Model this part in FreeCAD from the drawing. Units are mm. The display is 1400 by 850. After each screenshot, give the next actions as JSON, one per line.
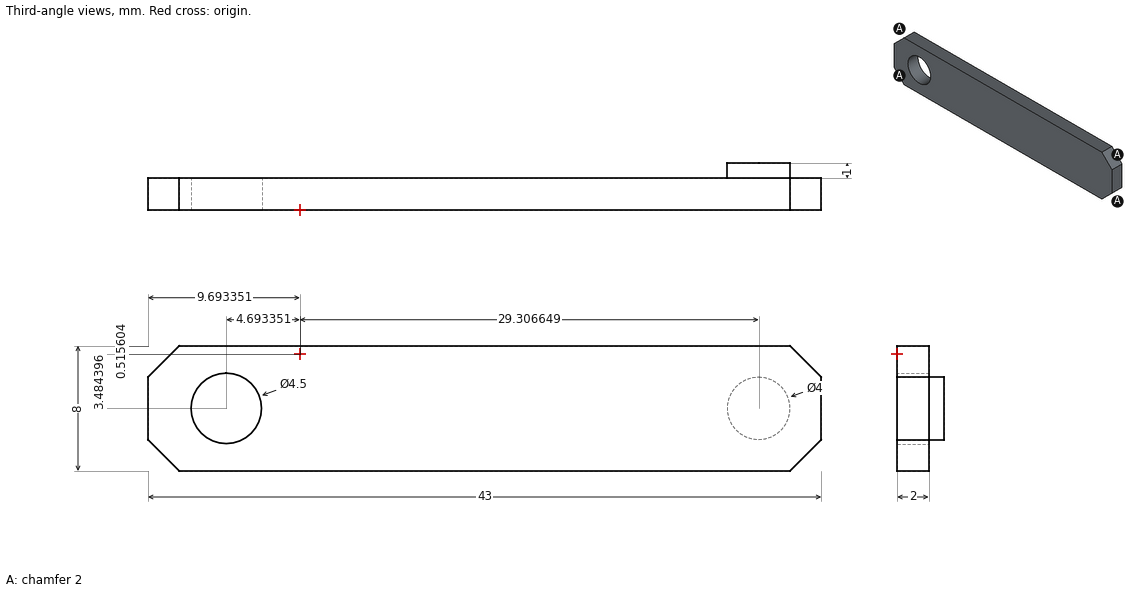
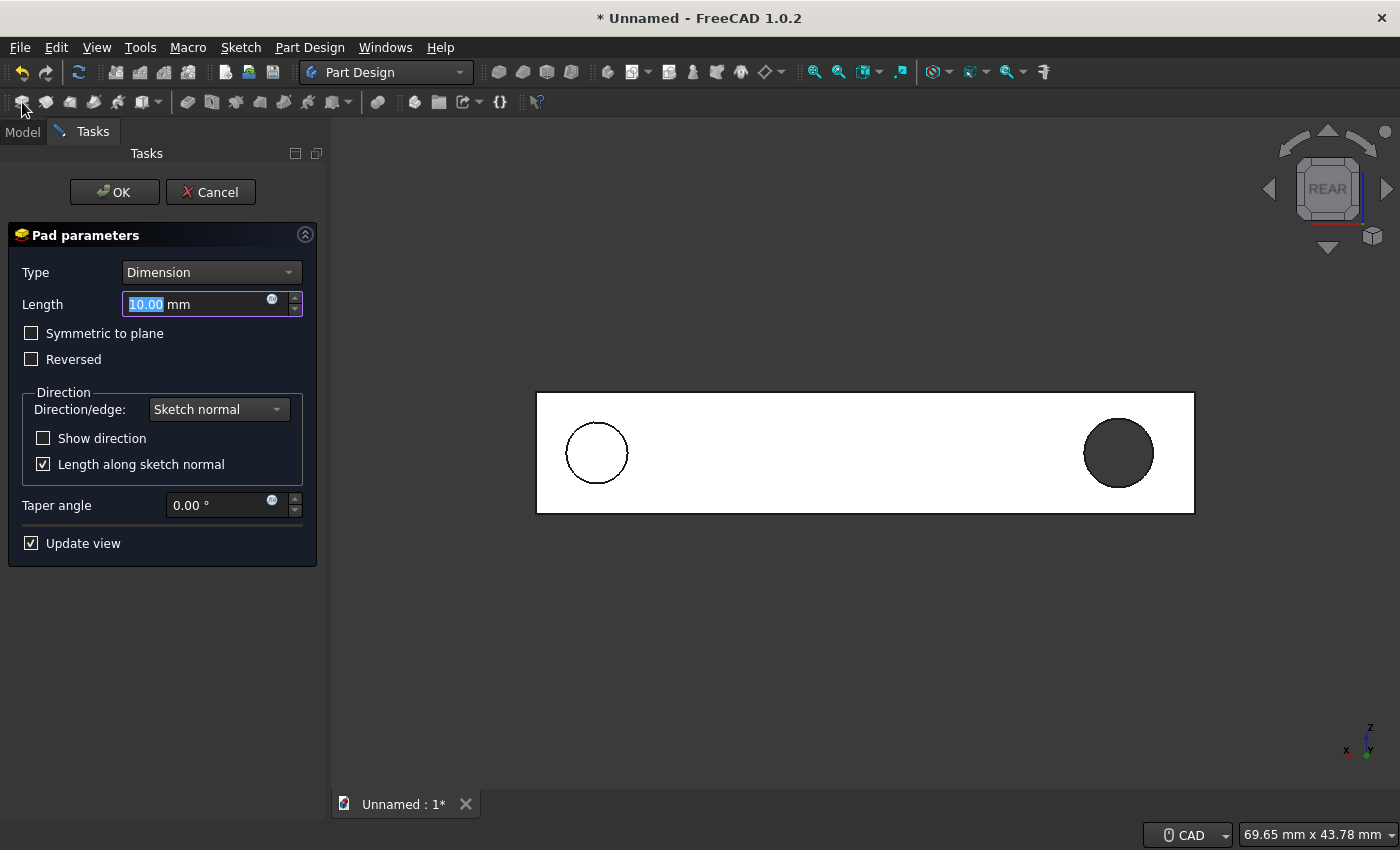
{"action": "type", "text": "1"}
{"action": "key", "text": "Tab"}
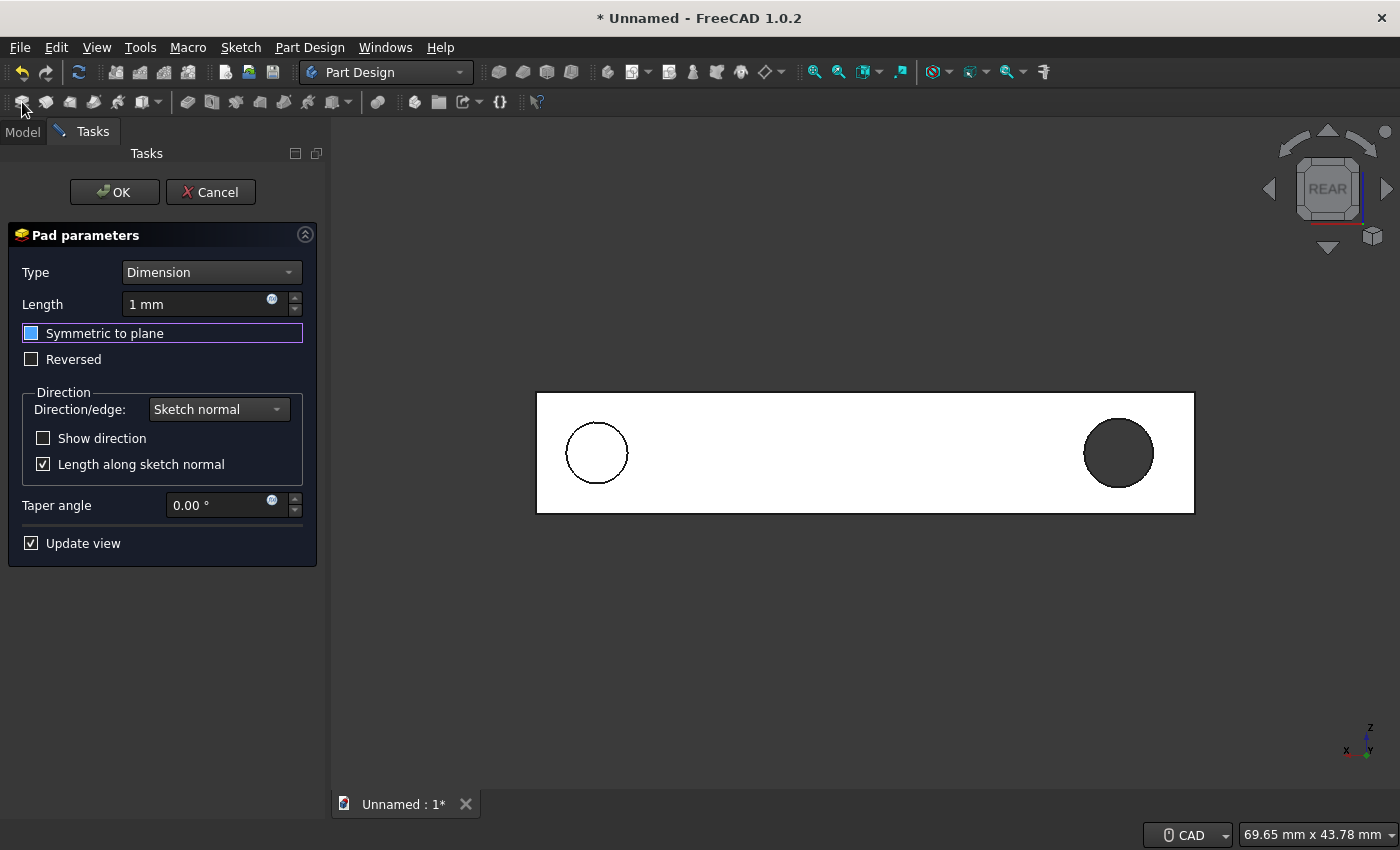
{"action": "left_click", "coordinate": [115, 192]}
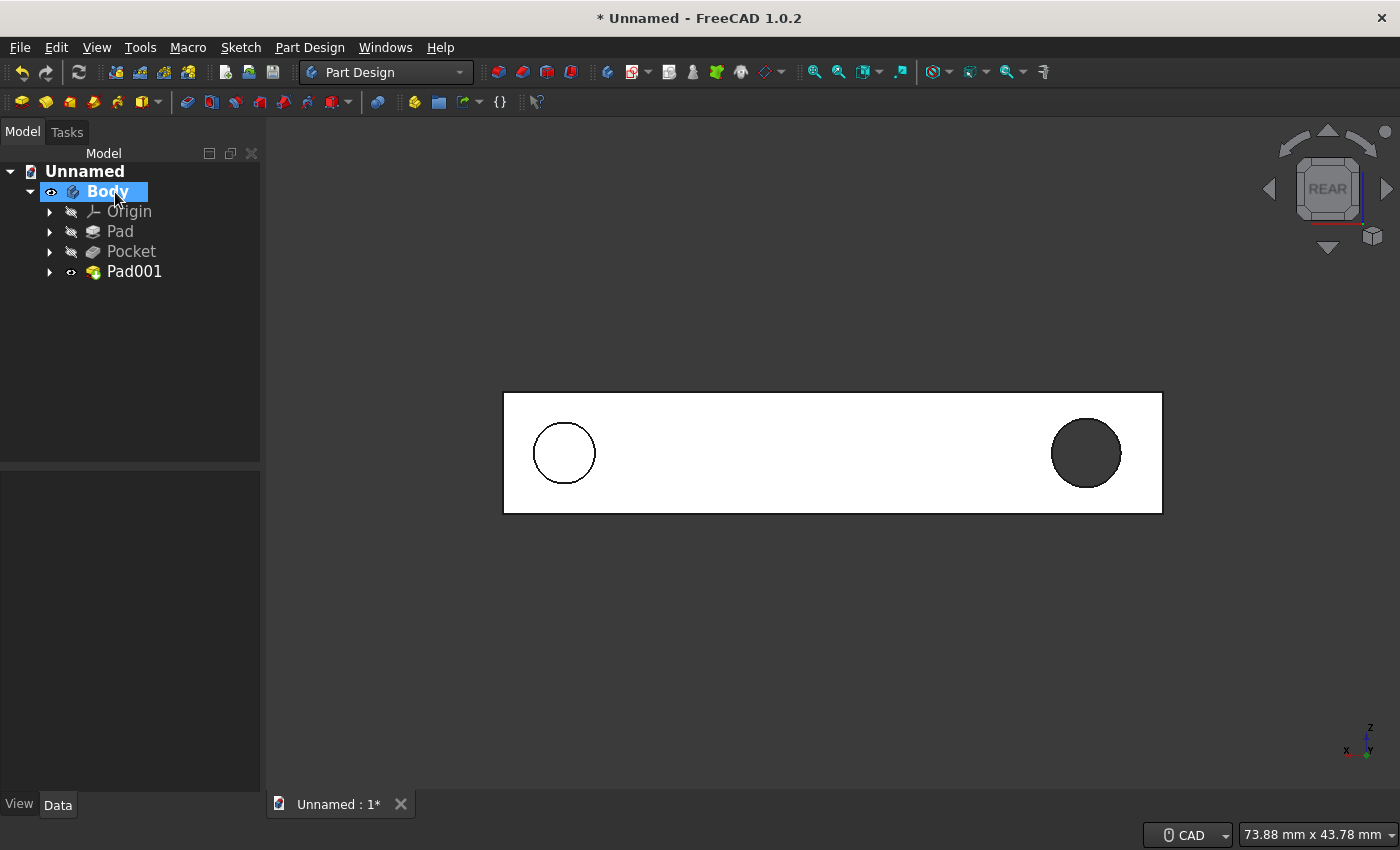
{"action": "key", "text": "0"}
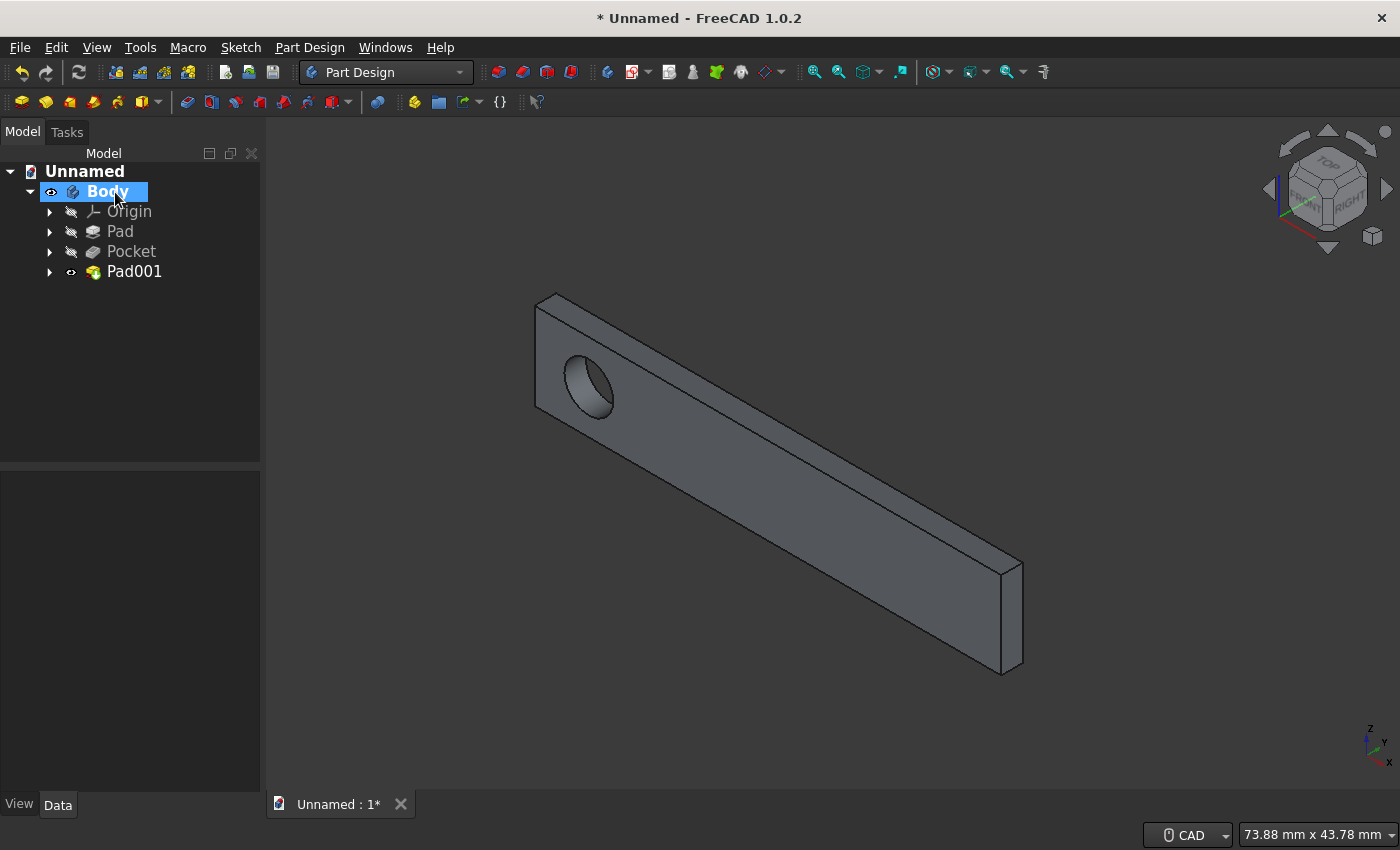
{"action": "left_click", "coordinate": [1012, 568]}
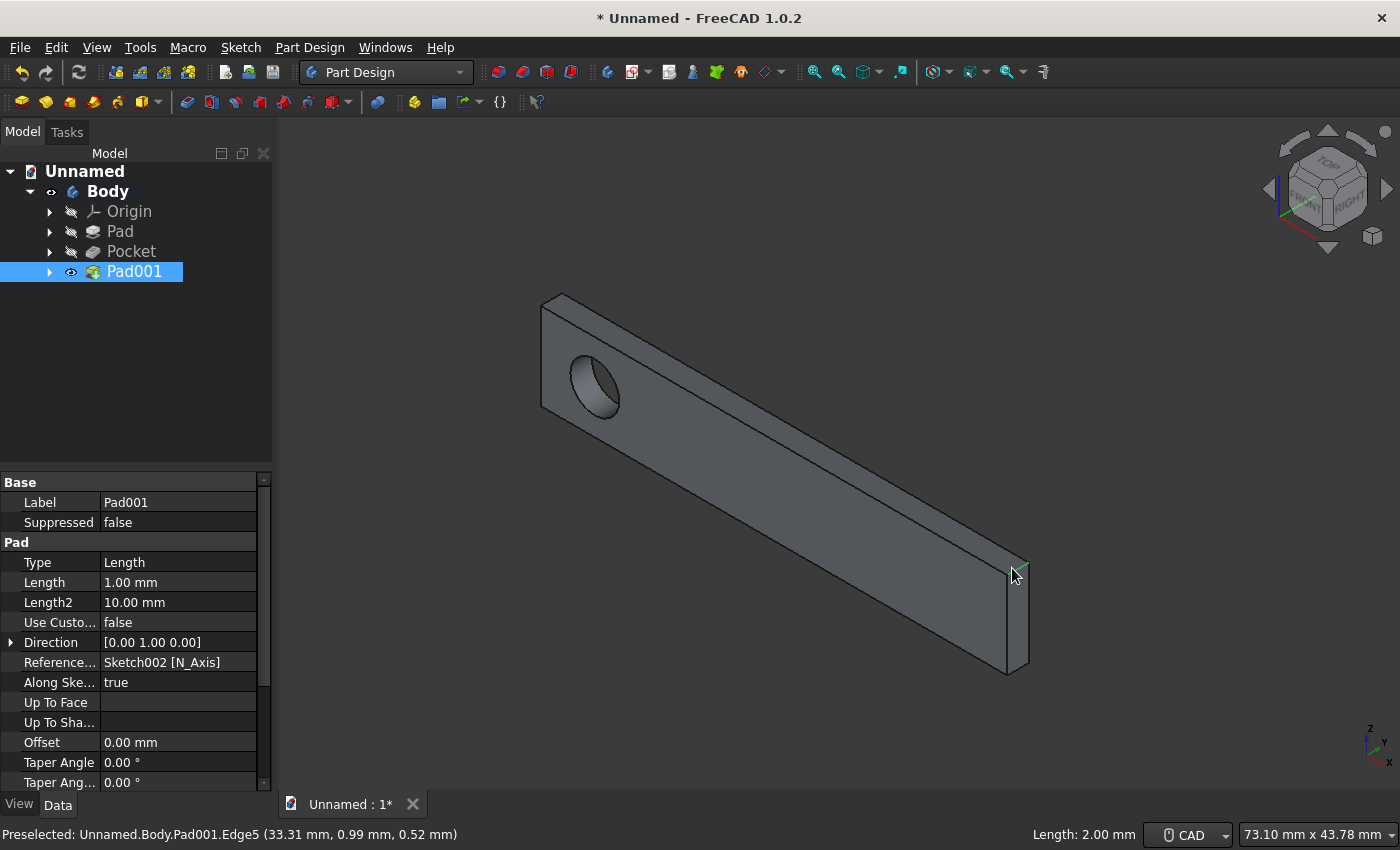
{"action": "key", "text": "2"}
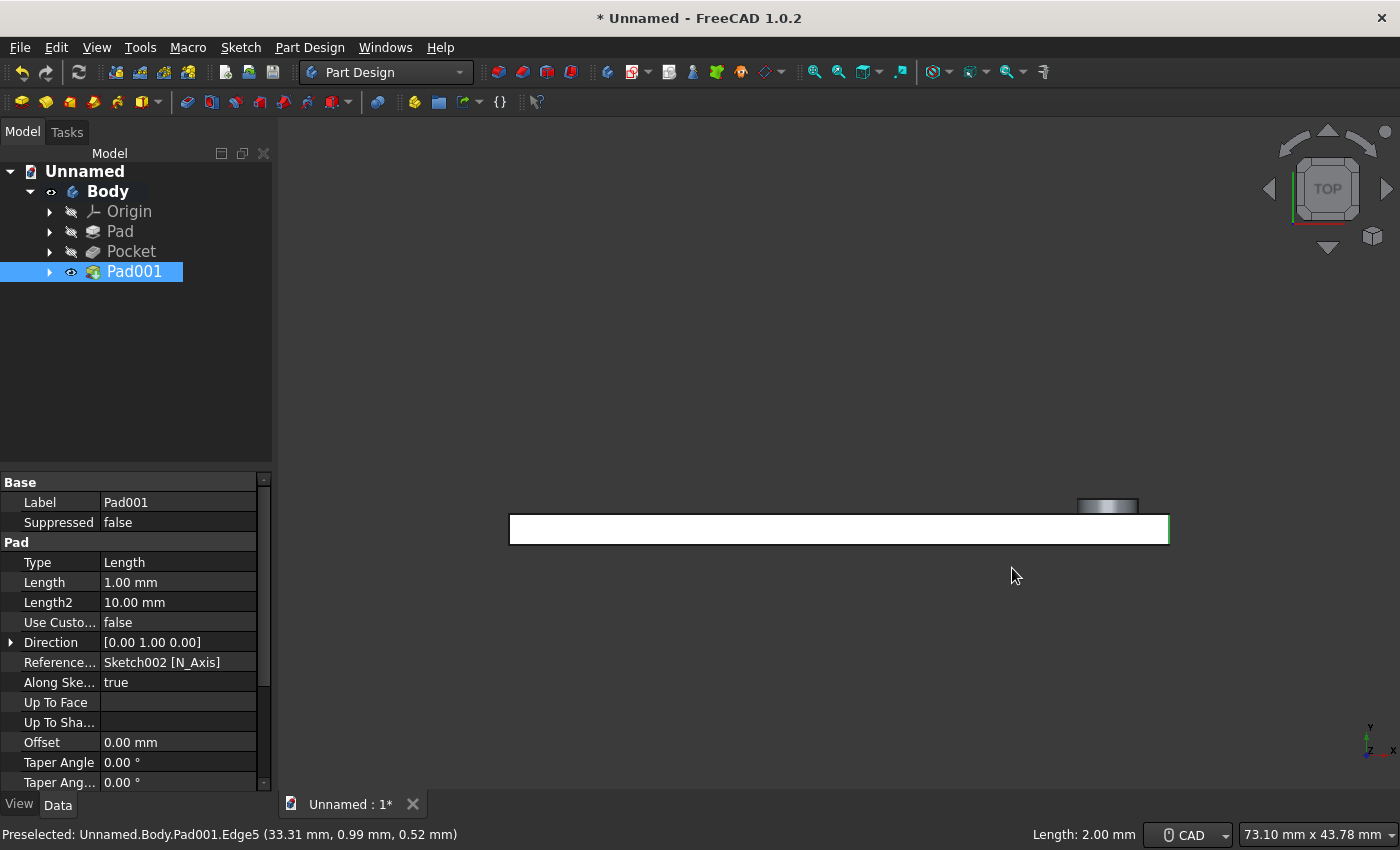
{"action": "left_click", "coordinate": [509, 529], "text": "ctrl"}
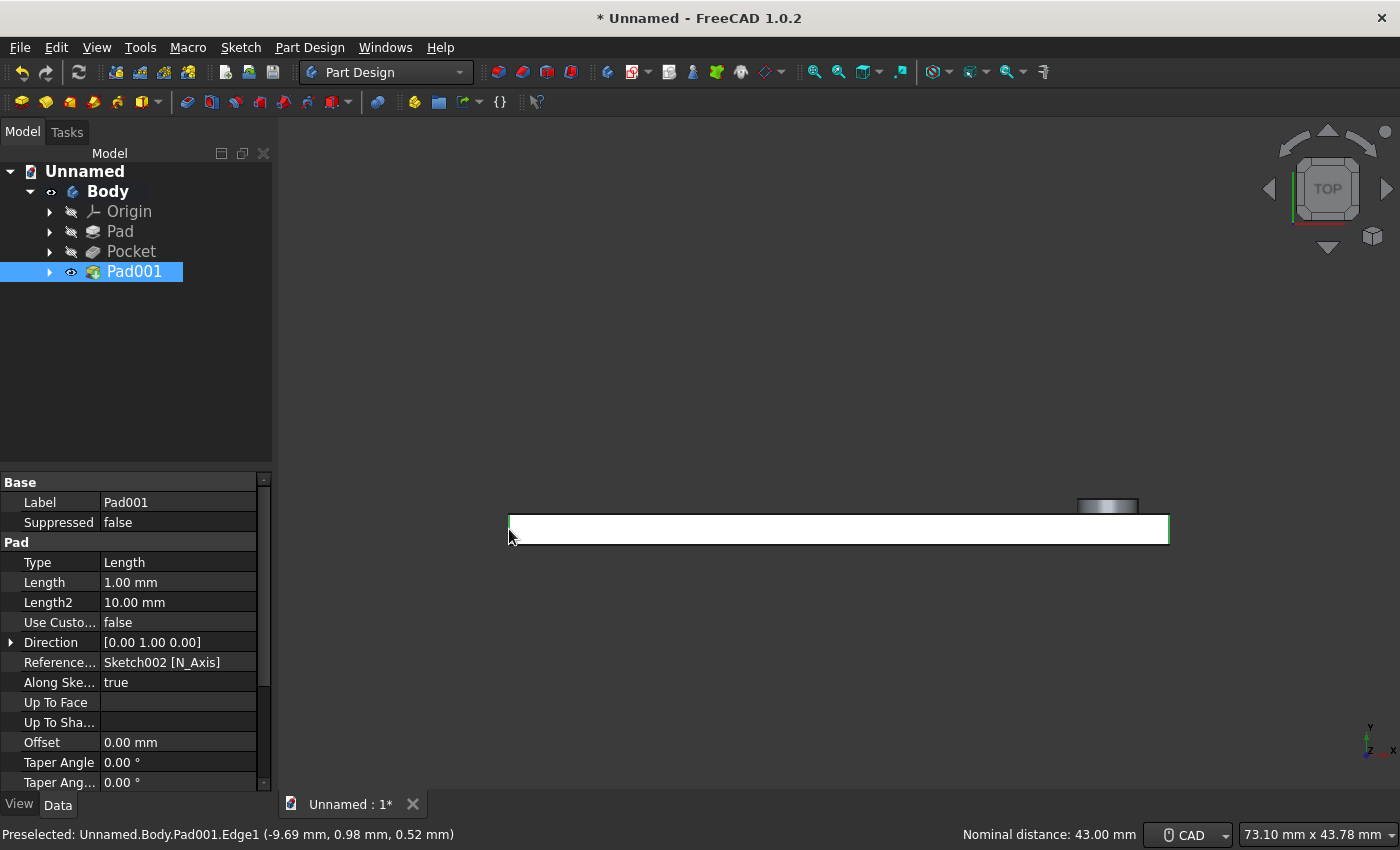
{"action": "key", "text": "1"}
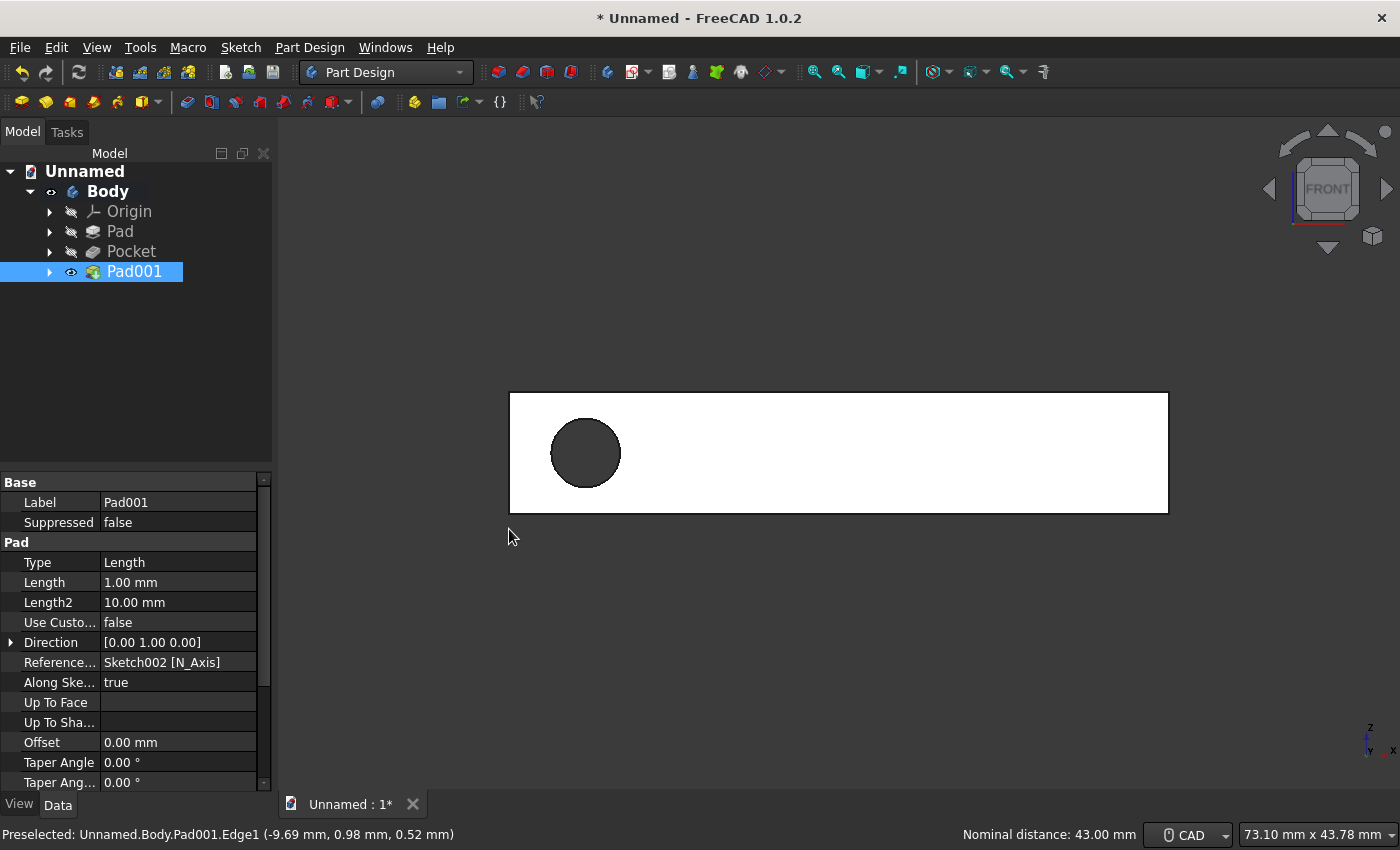
{"action": "key", "text": "3"}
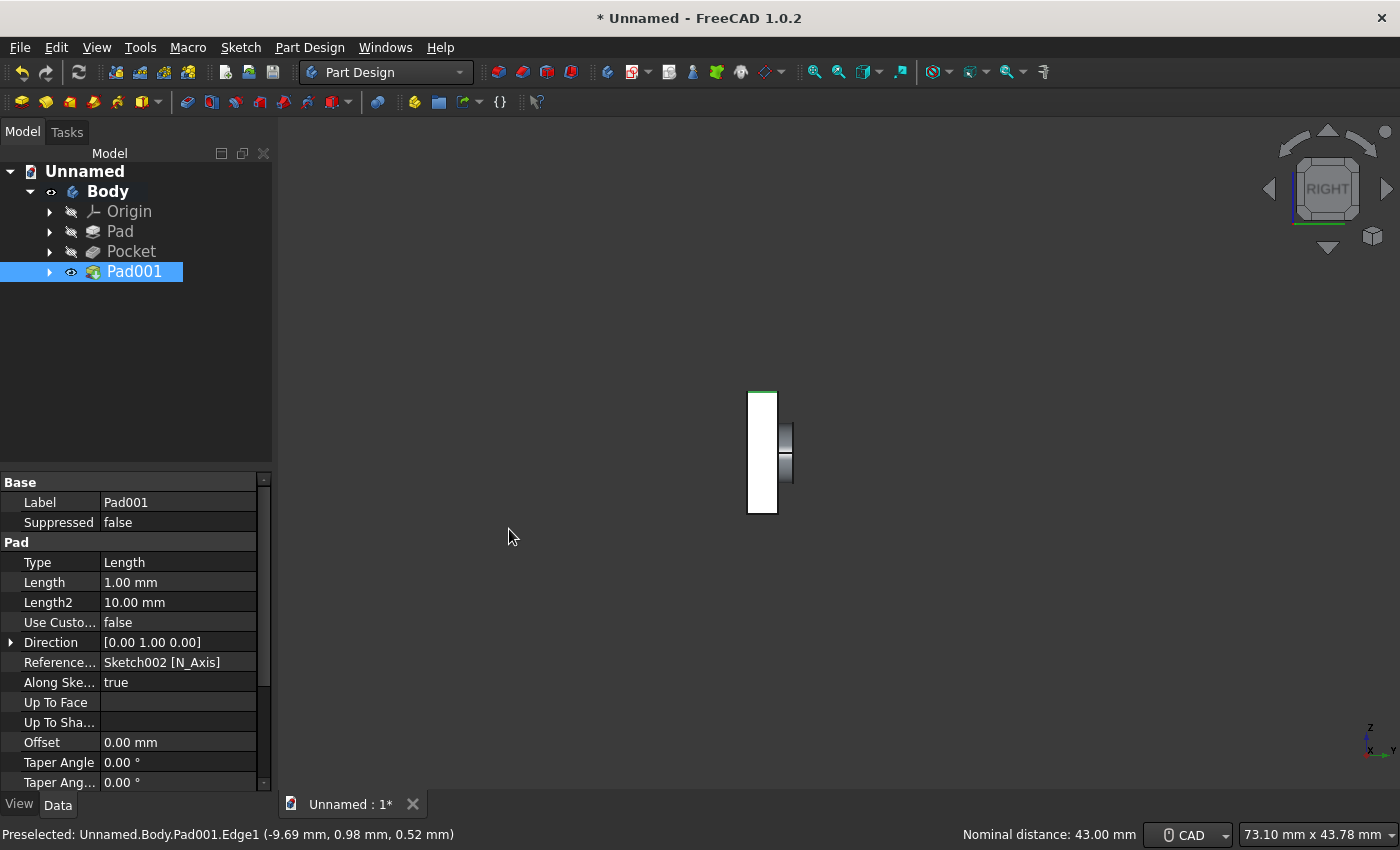
{"action": "left_click", "coordinate": [816, 72]}